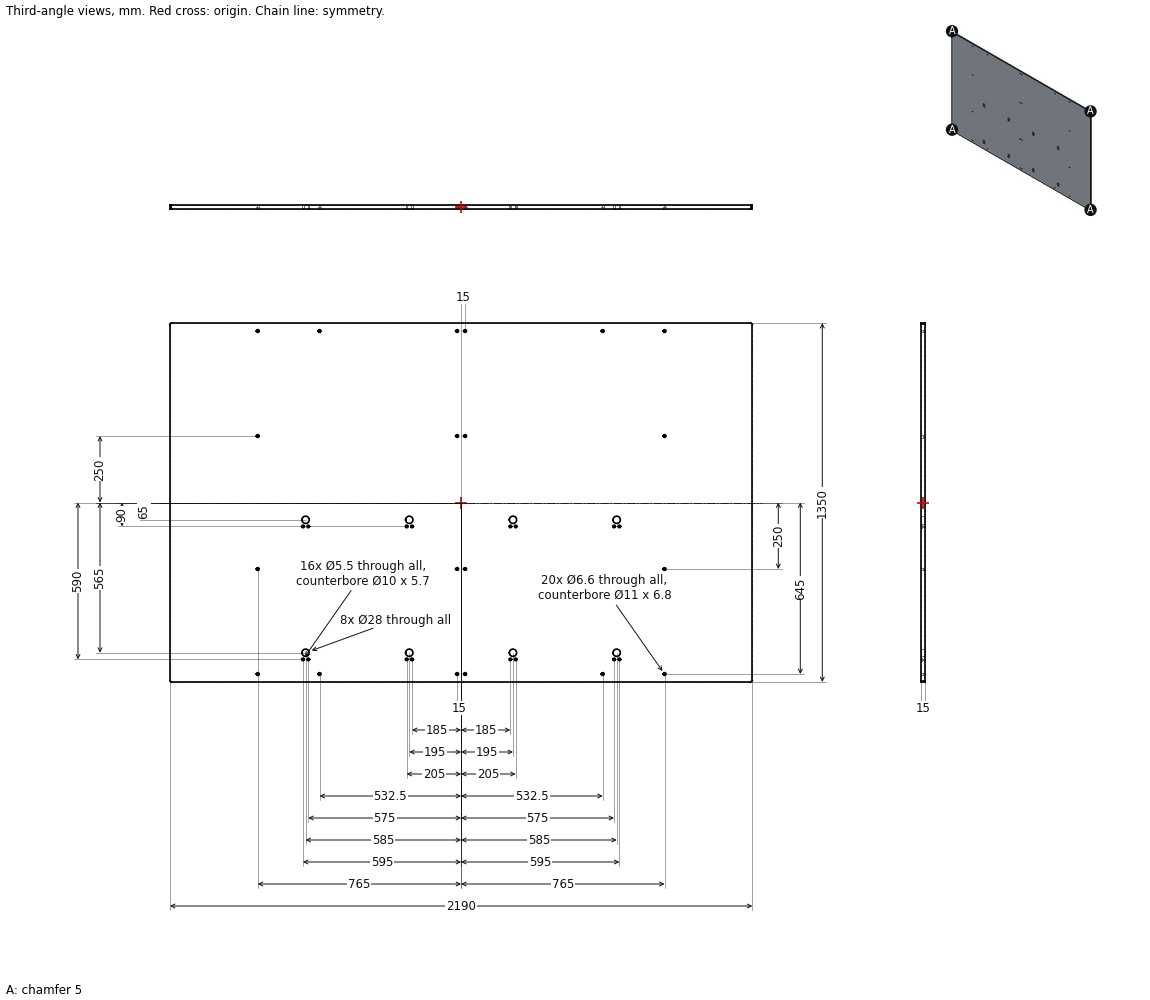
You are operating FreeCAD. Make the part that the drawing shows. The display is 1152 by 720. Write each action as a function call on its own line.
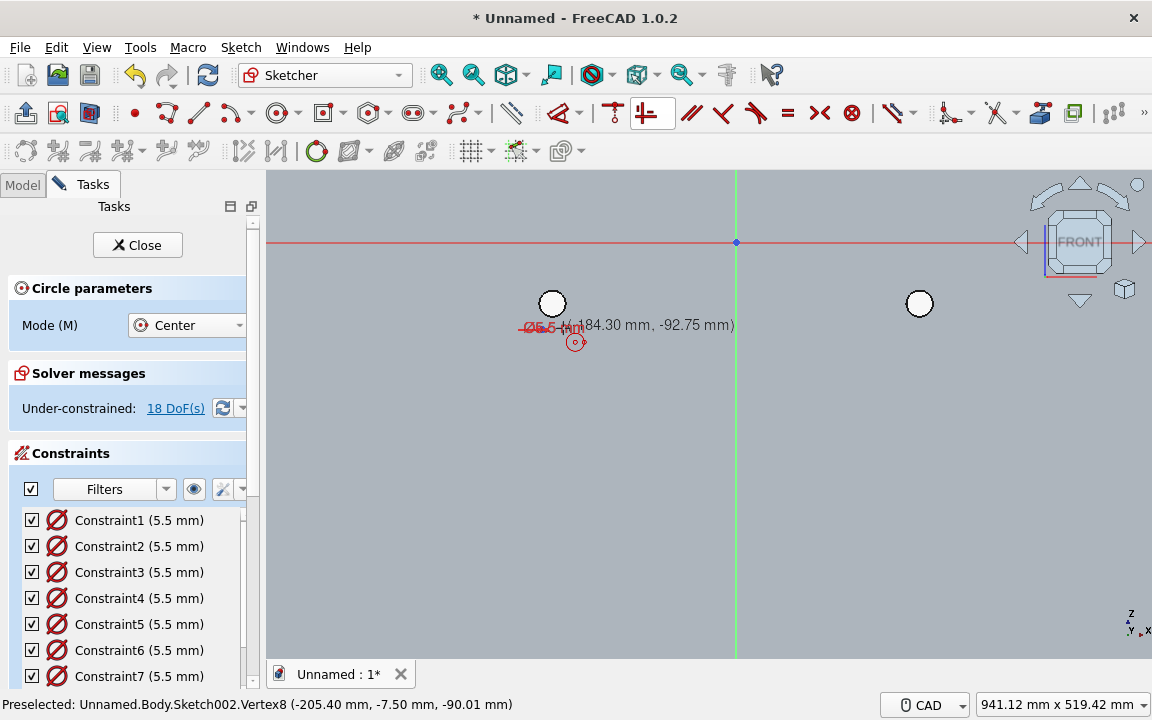
click(562, 327)
move(564, 325)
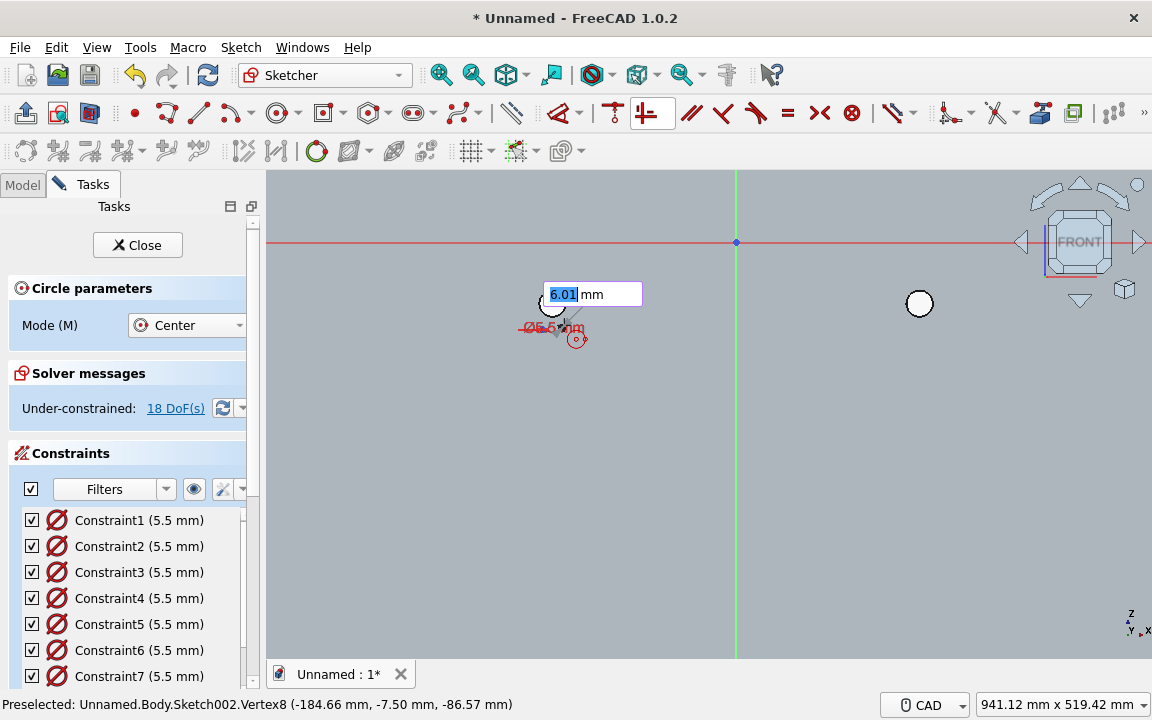
text(5.5)
key(Return)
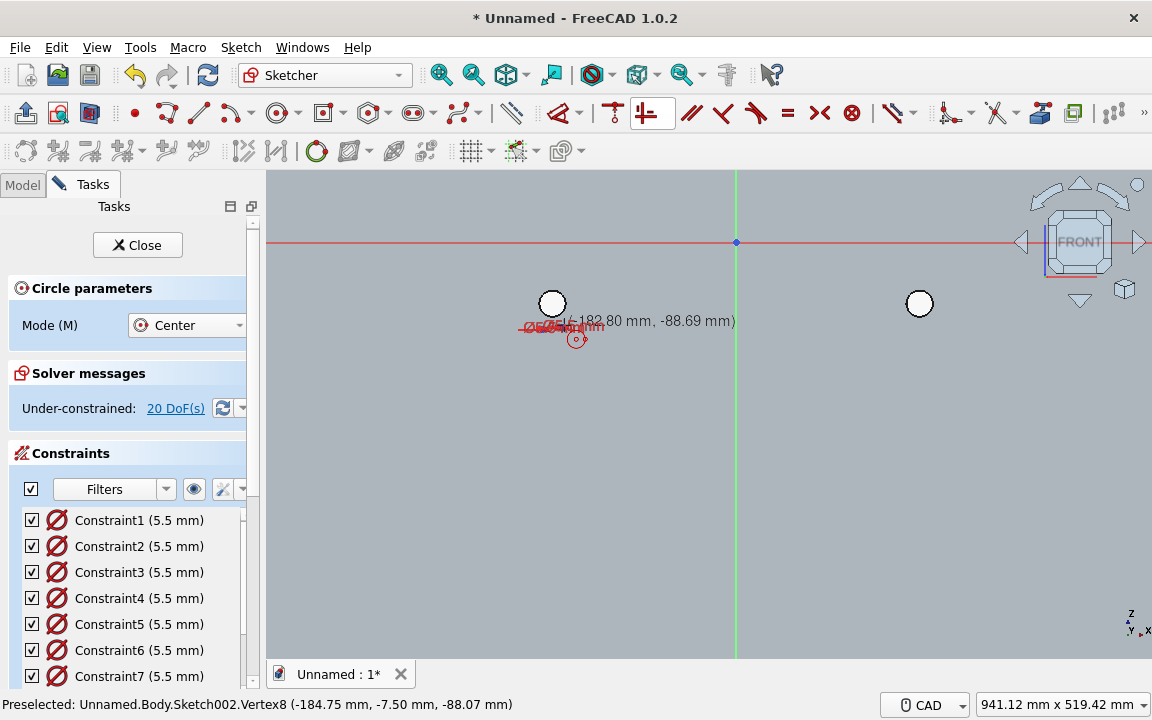
scroll(910, 327, up, 11)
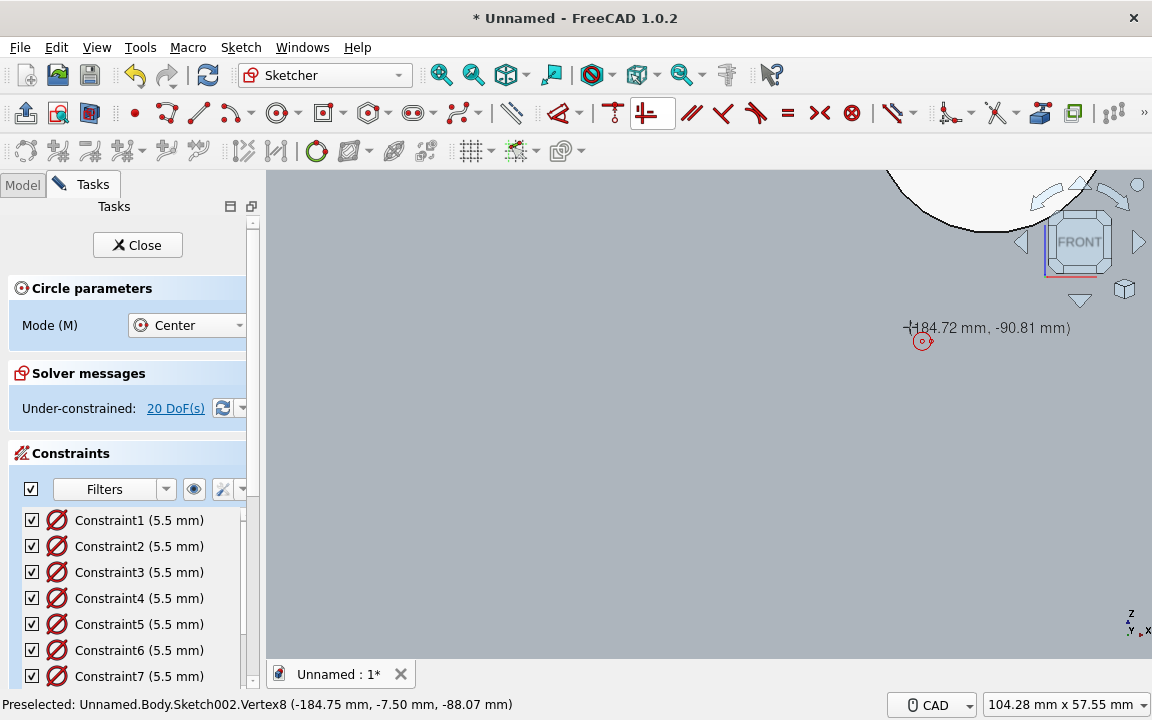
scroll(709, 327, down, 15)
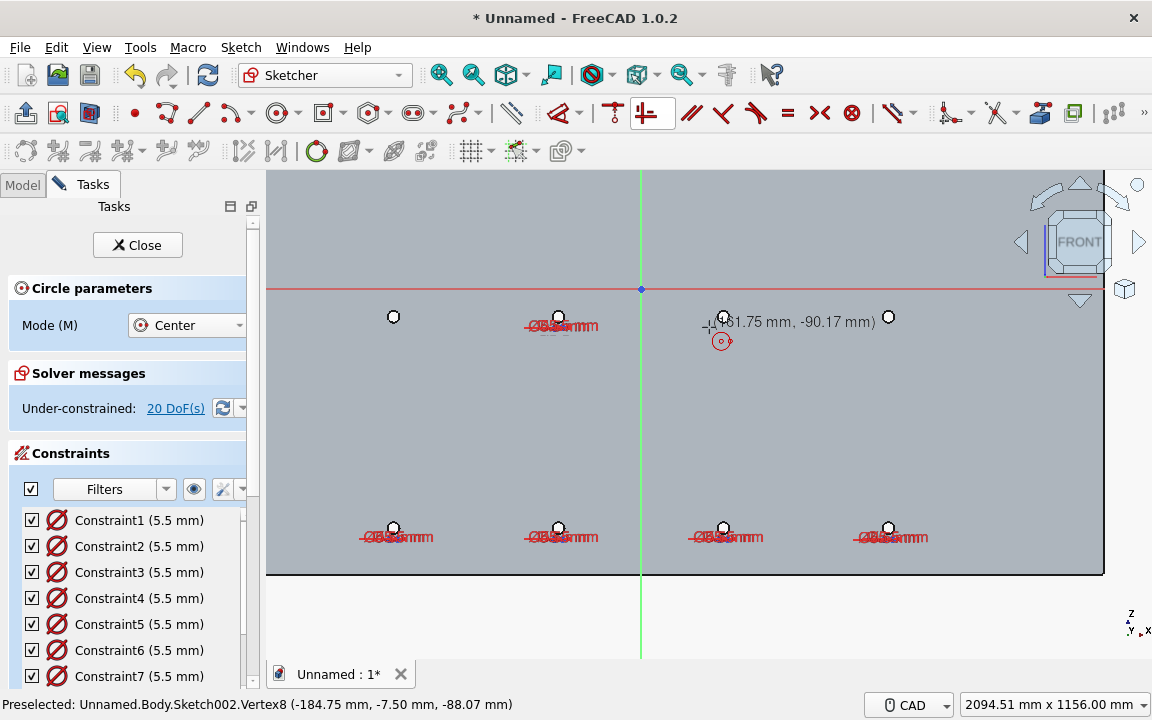
click(719, 327)
move(720, 326)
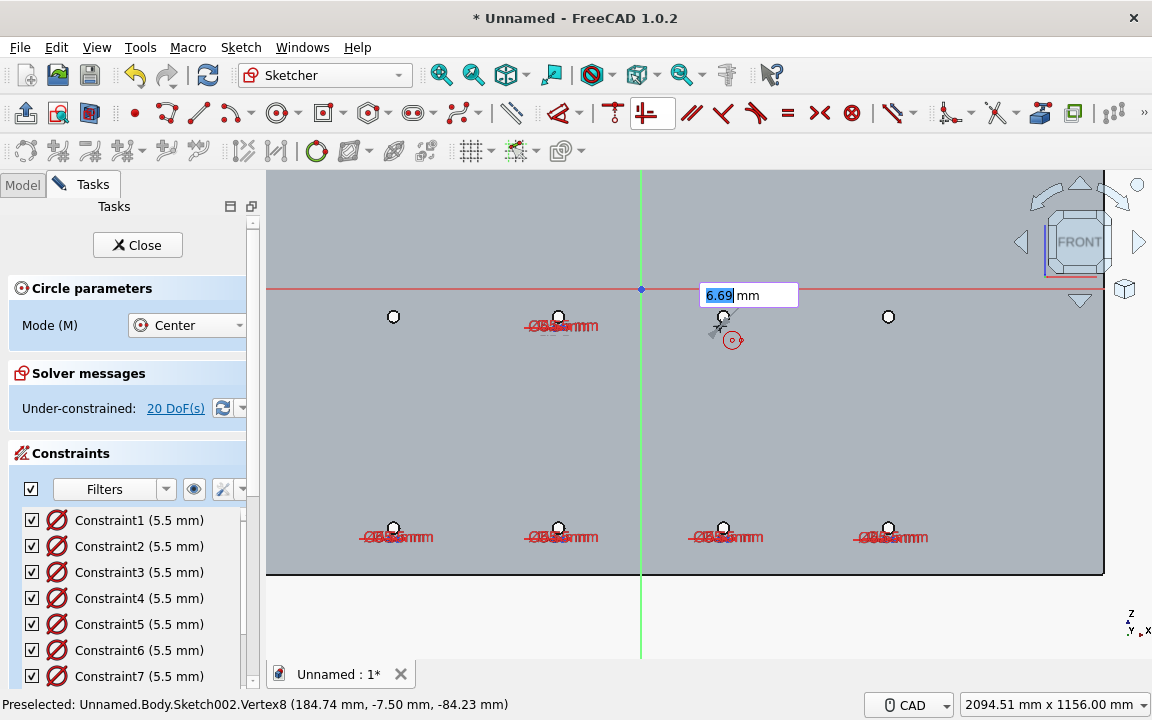
text(5.5)
key(Return)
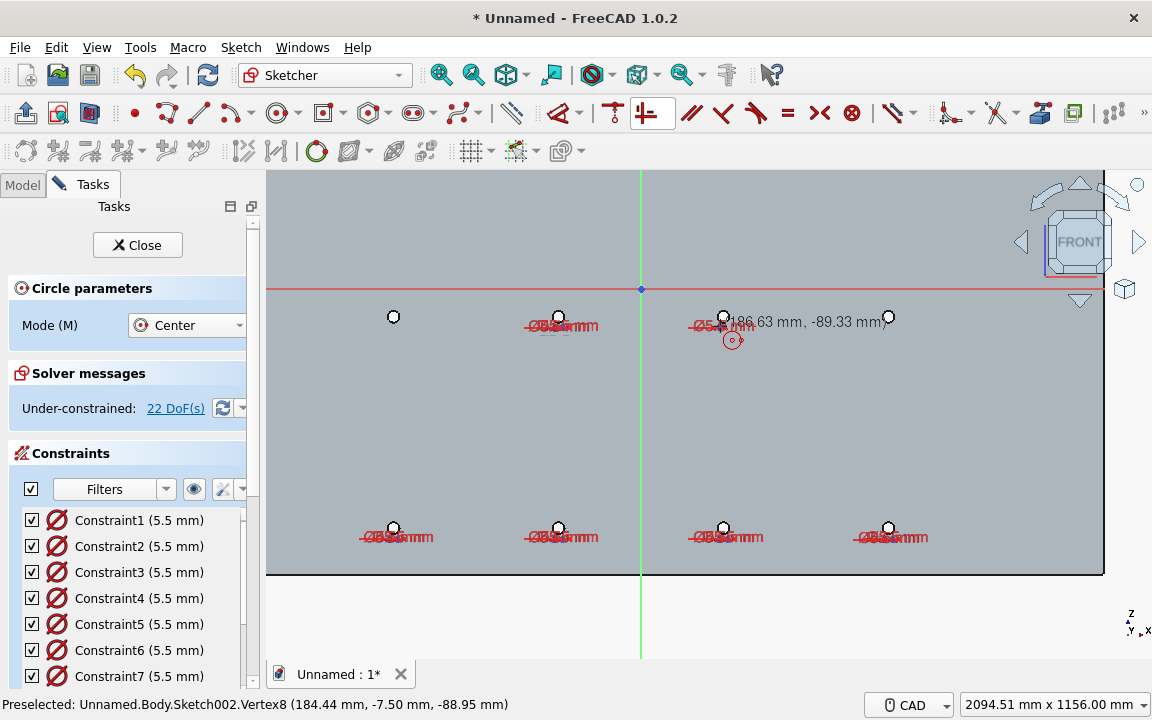
scroll(728, 327, up, 15)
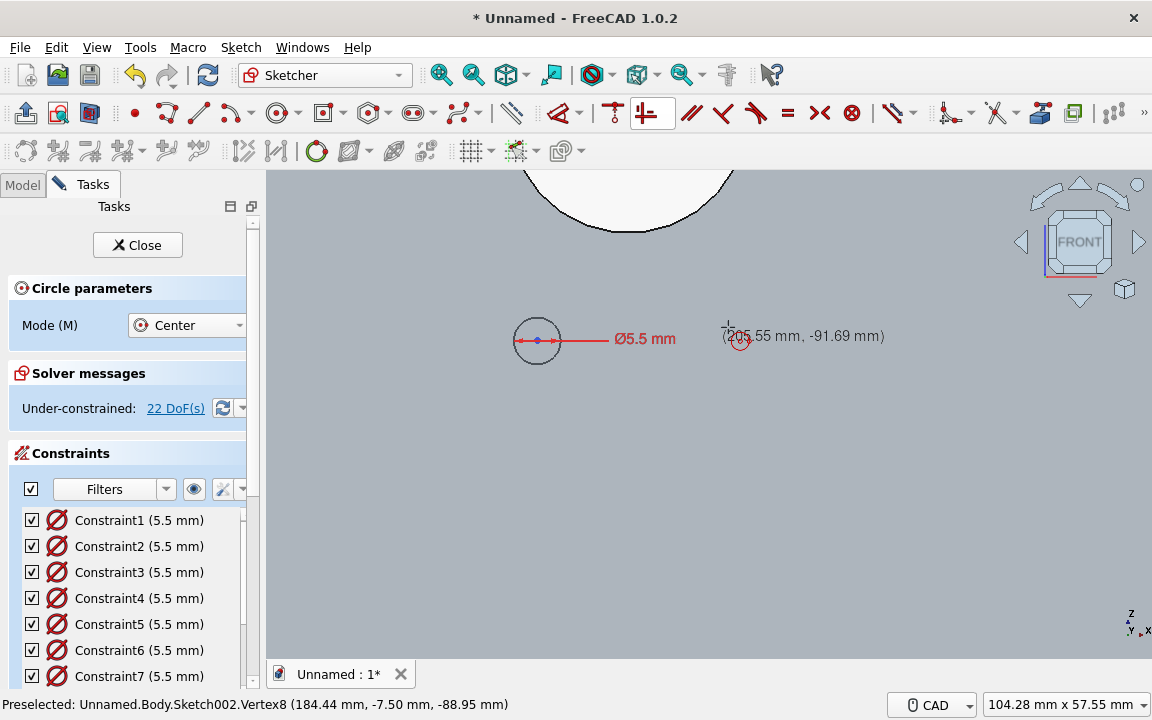
scroll(728, 327, down, 15)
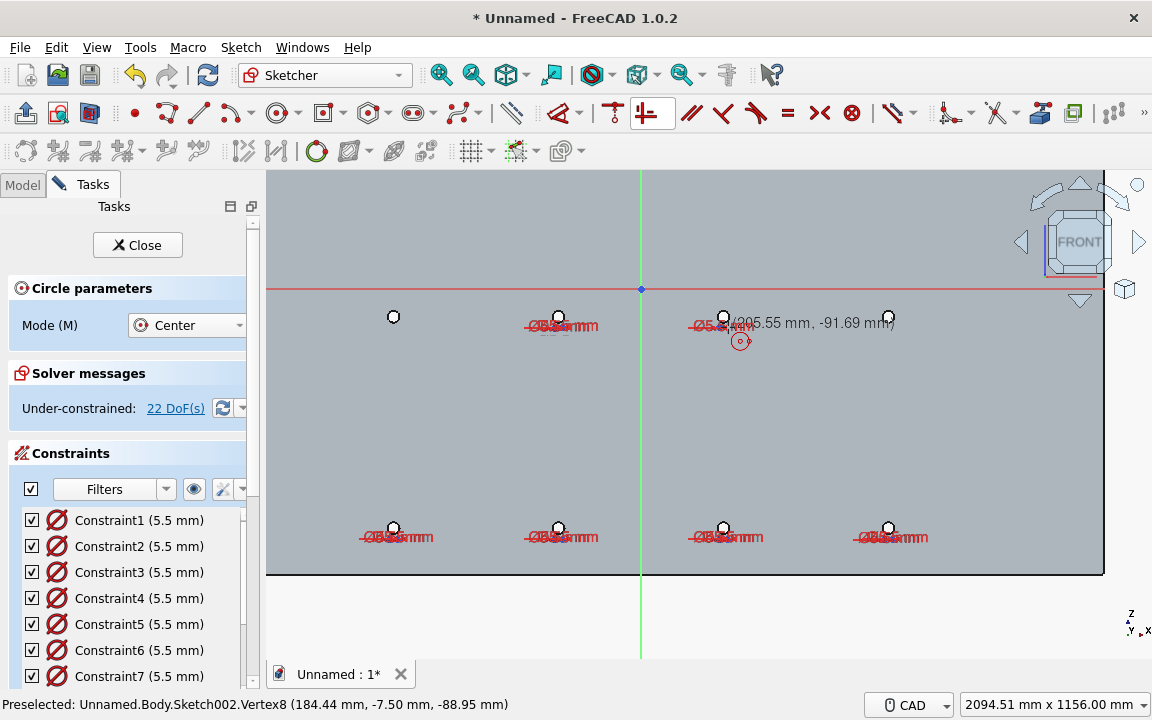
scroll(728, 327, up, 4)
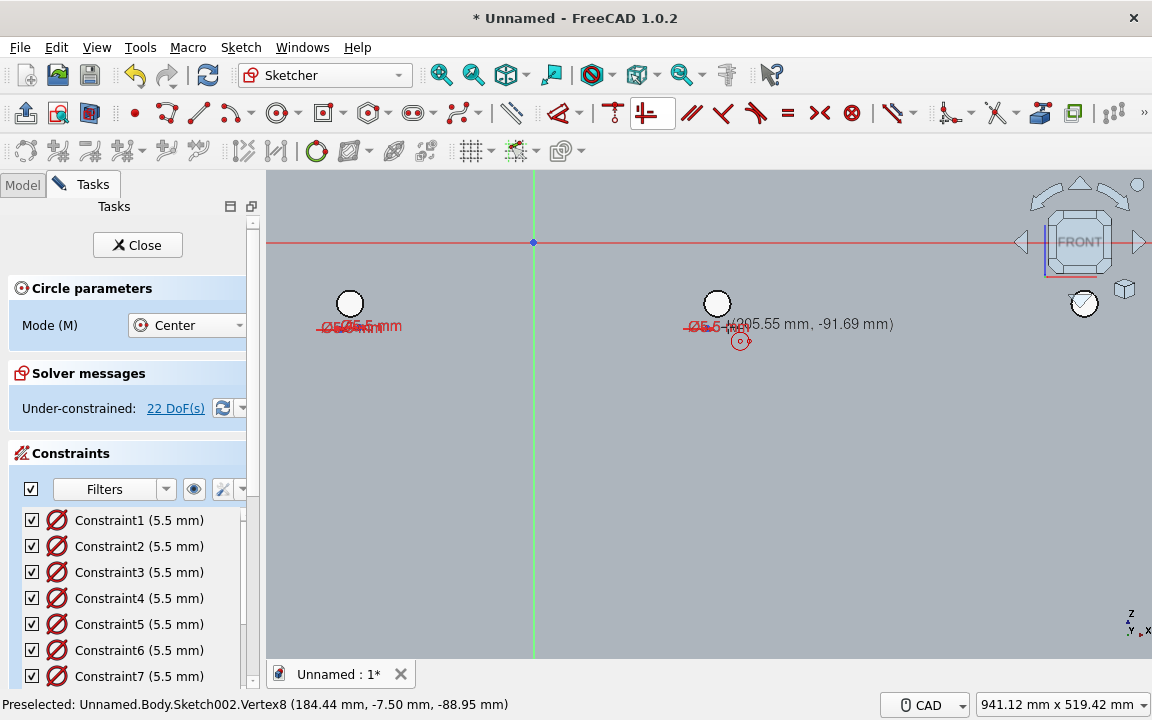
click(727, 327)
move(729, 325)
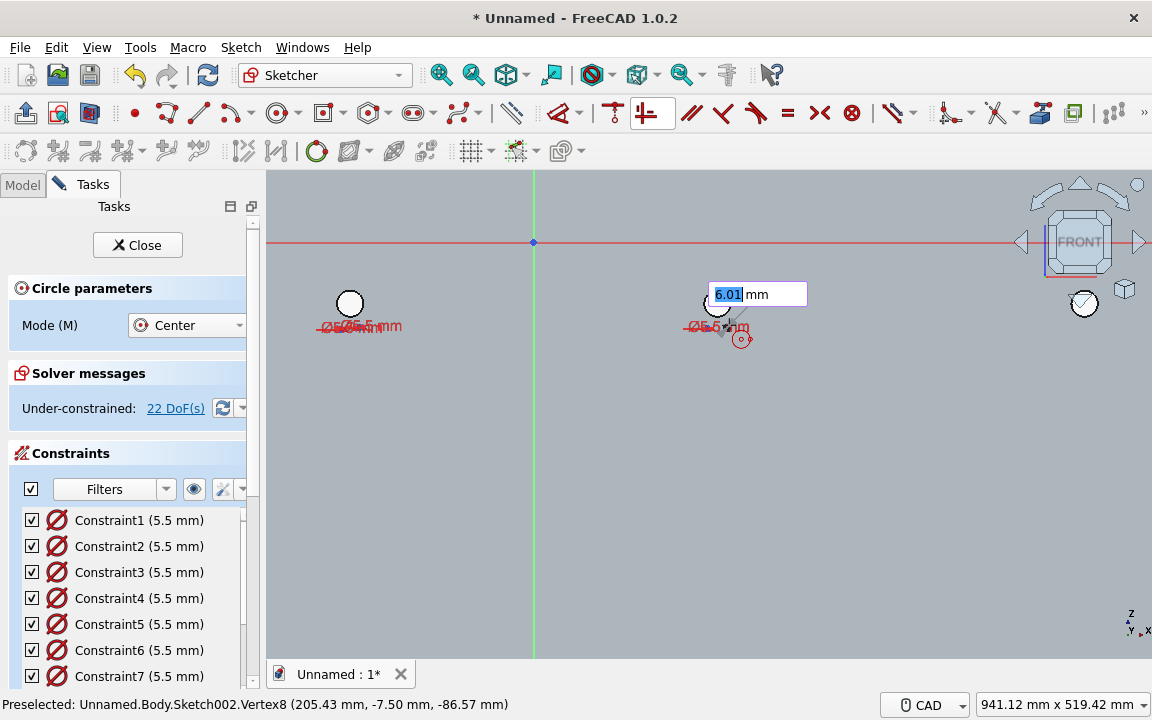
text(5.5)
key(Return)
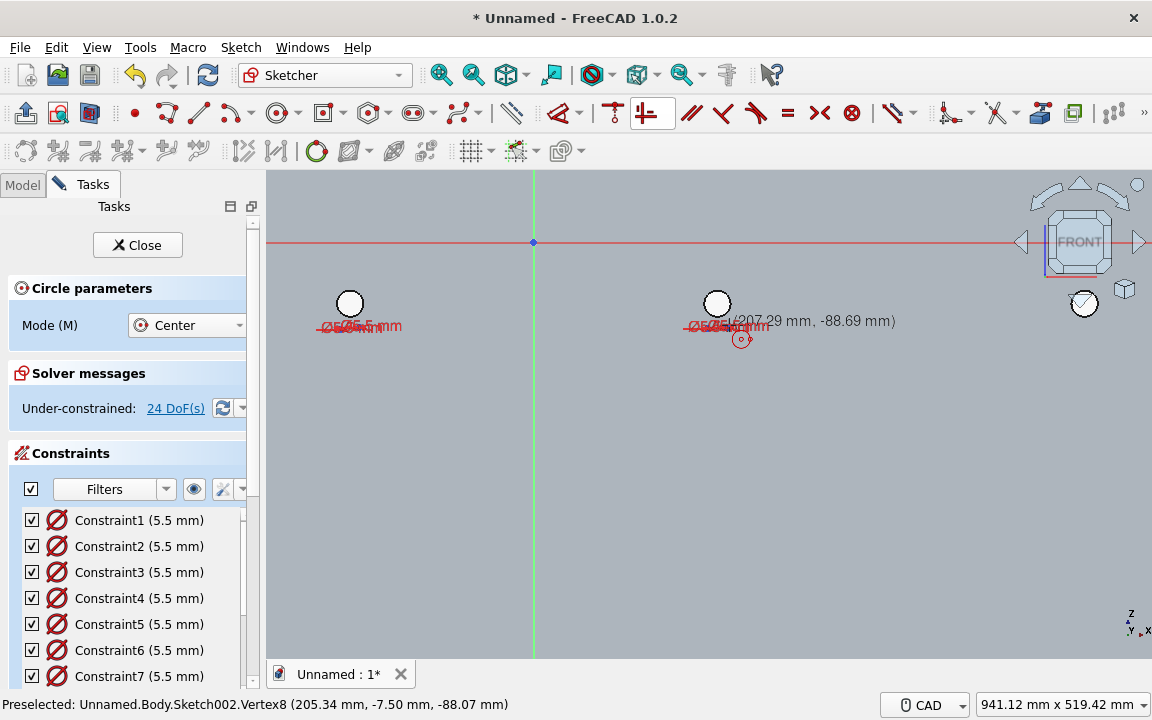
scroll(728, 327, down, 4)